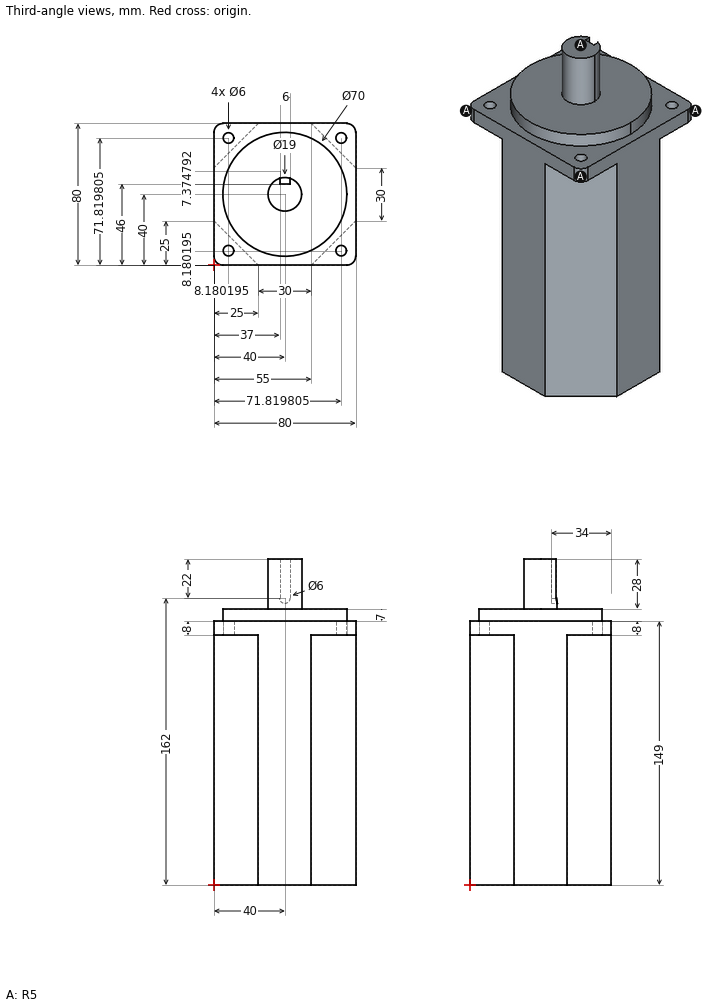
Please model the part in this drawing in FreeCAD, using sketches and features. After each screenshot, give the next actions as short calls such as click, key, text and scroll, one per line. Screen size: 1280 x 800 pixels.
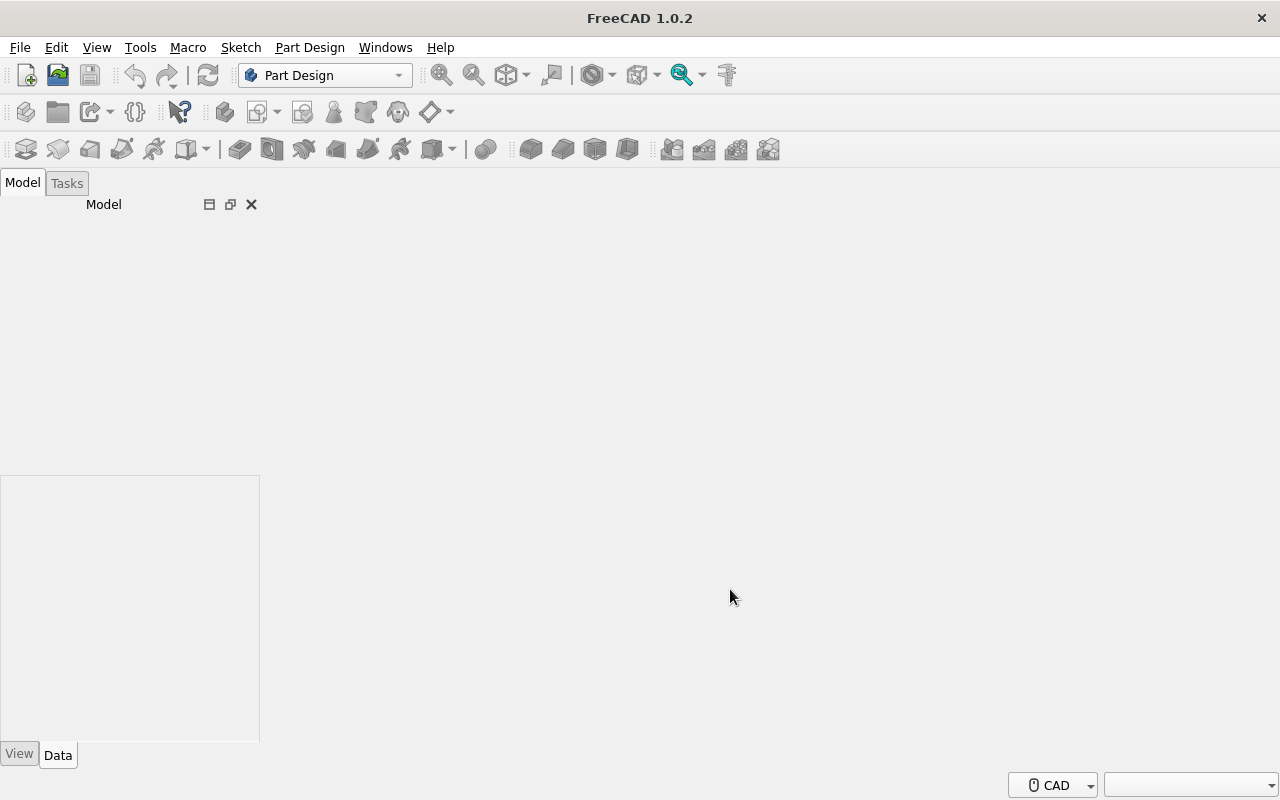
key(ctrl+n)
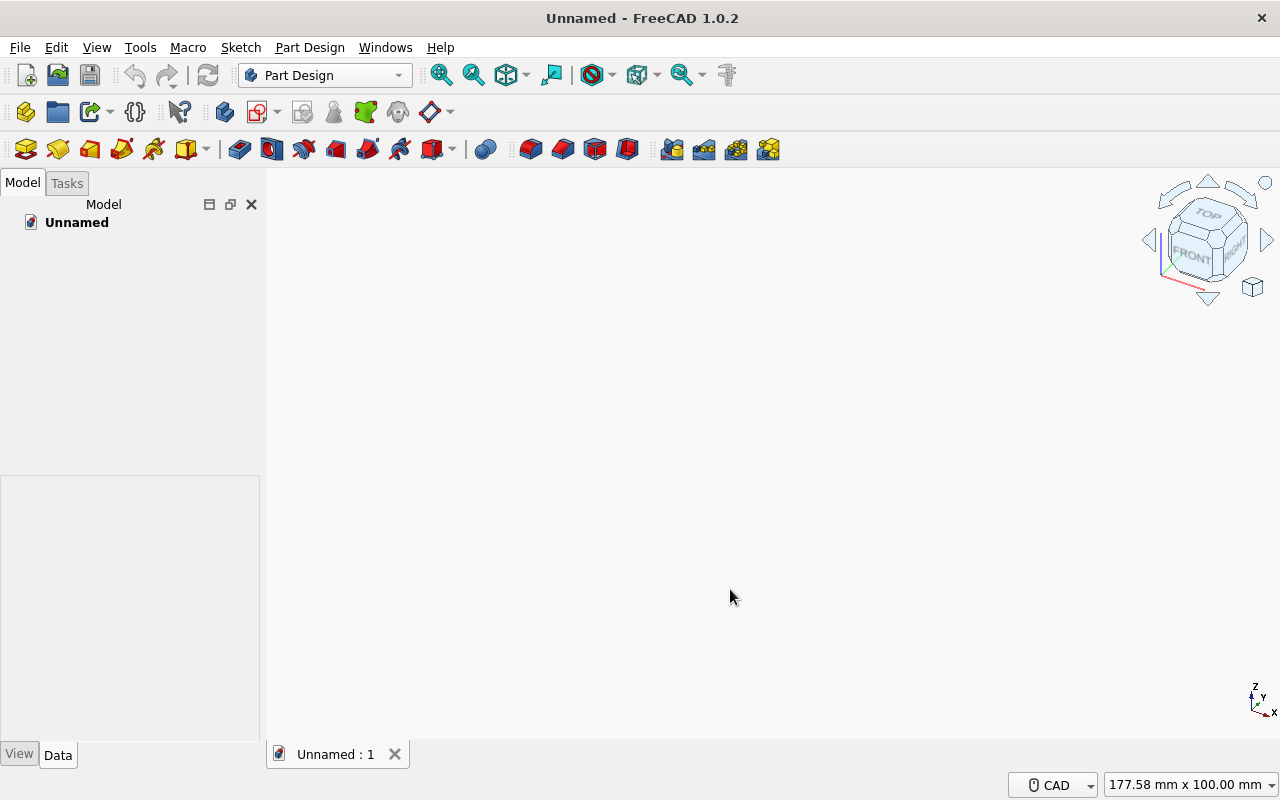
click(258, 112)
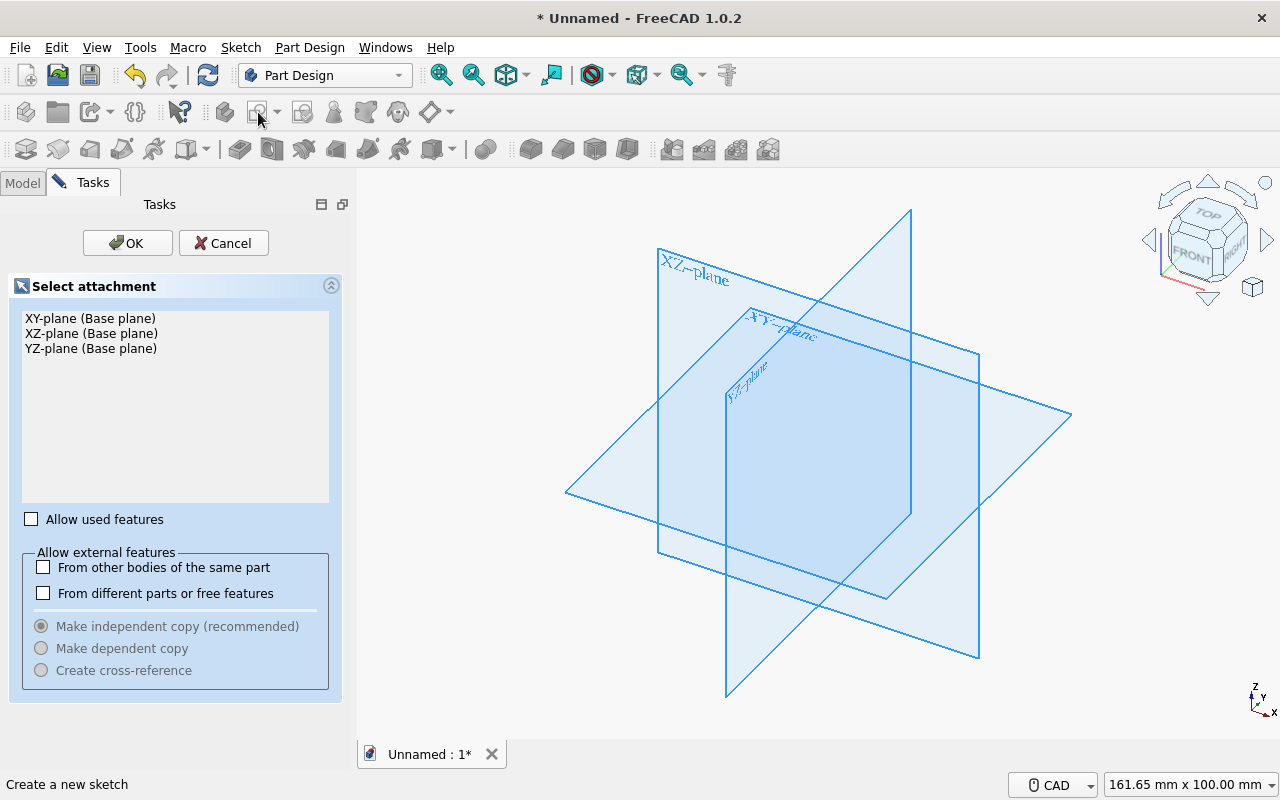
click(82, 318)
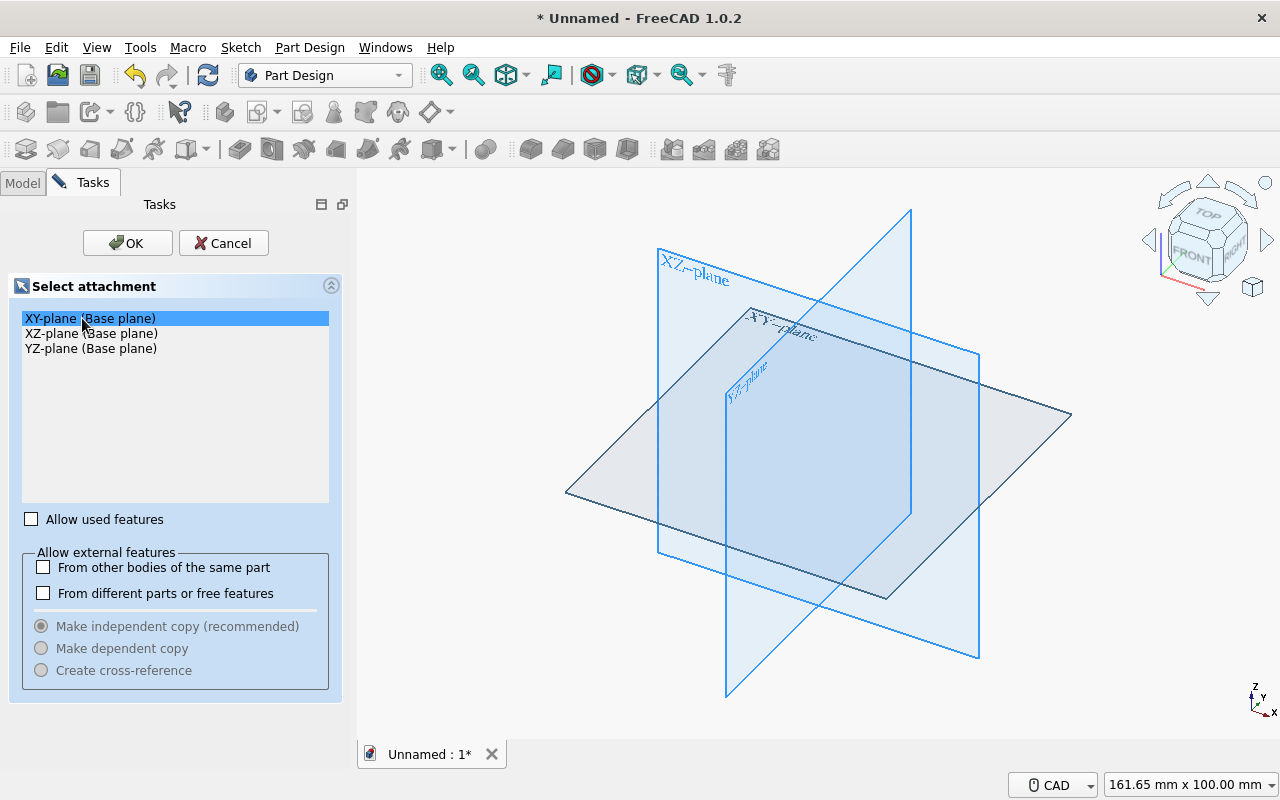
click(128, 243)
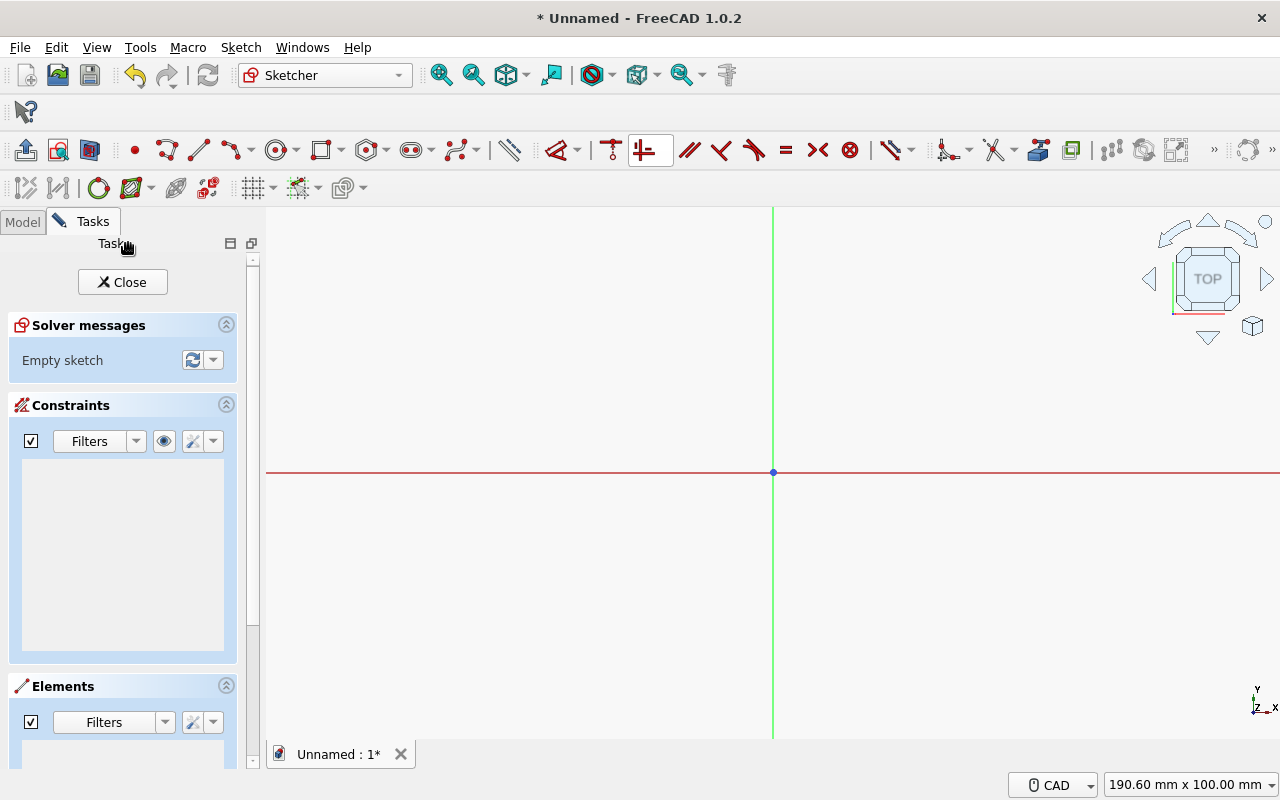
scroll(294, 711, down, 2)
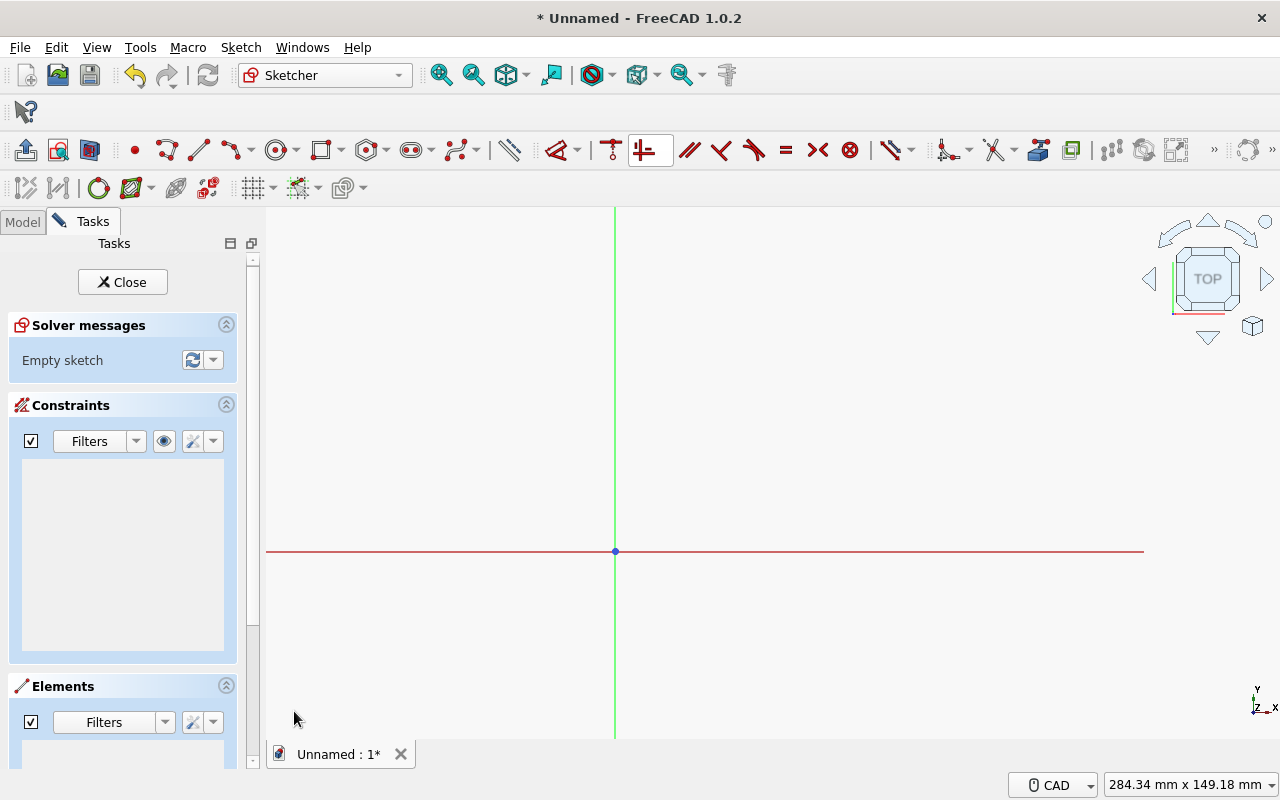
key(g)
key(m)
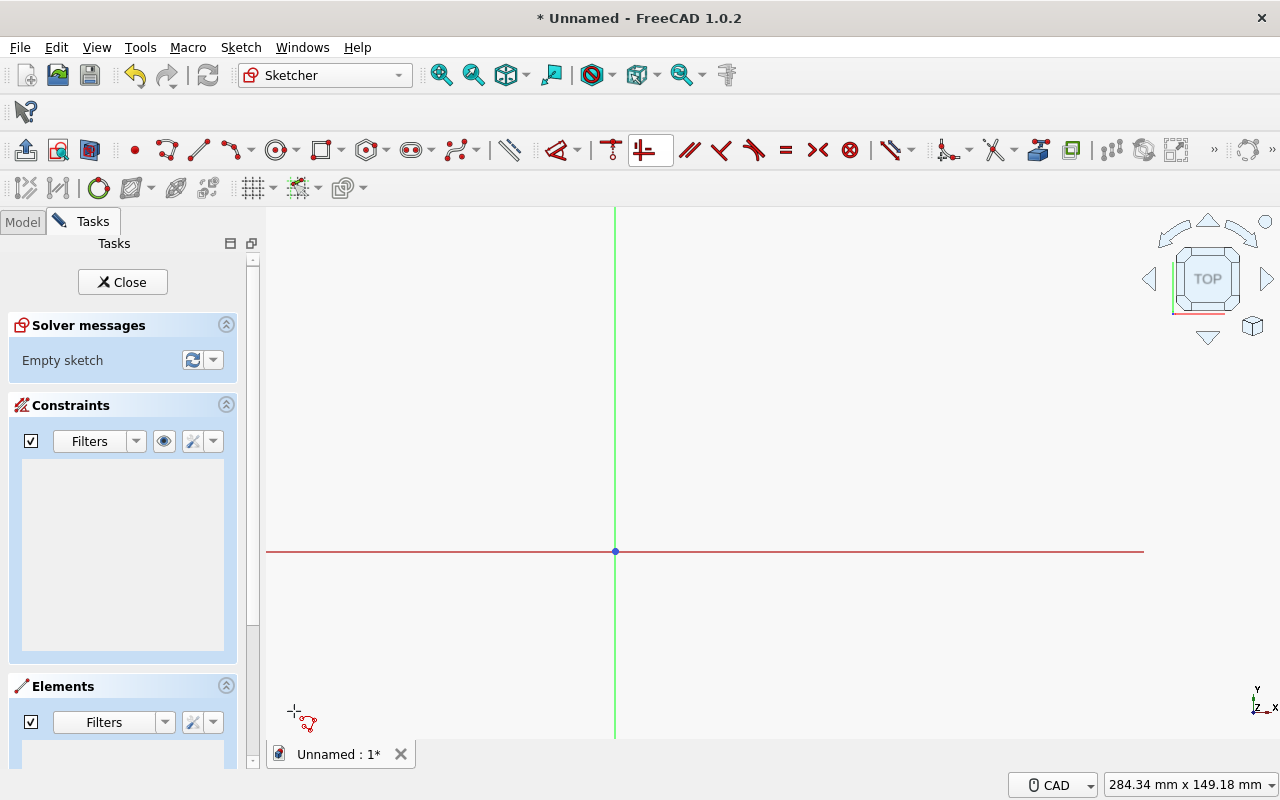
click(615, 463)
click(704, 552)
click(811, 543)
click(900, 463)
click(900, 356)
click(811, 266)
click(704, 266)
click(624, 356)
click(615, 464)
key(Escape)
key(Escape)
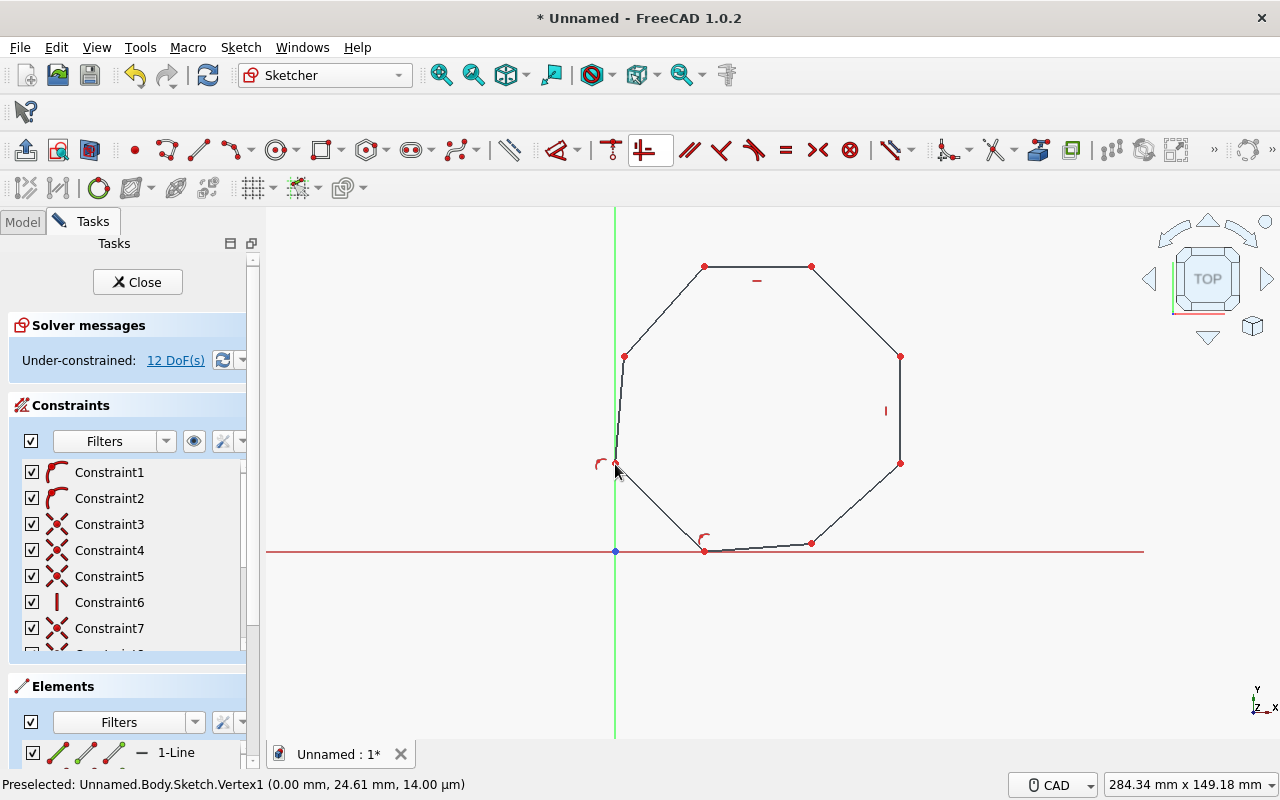
click(736, 549)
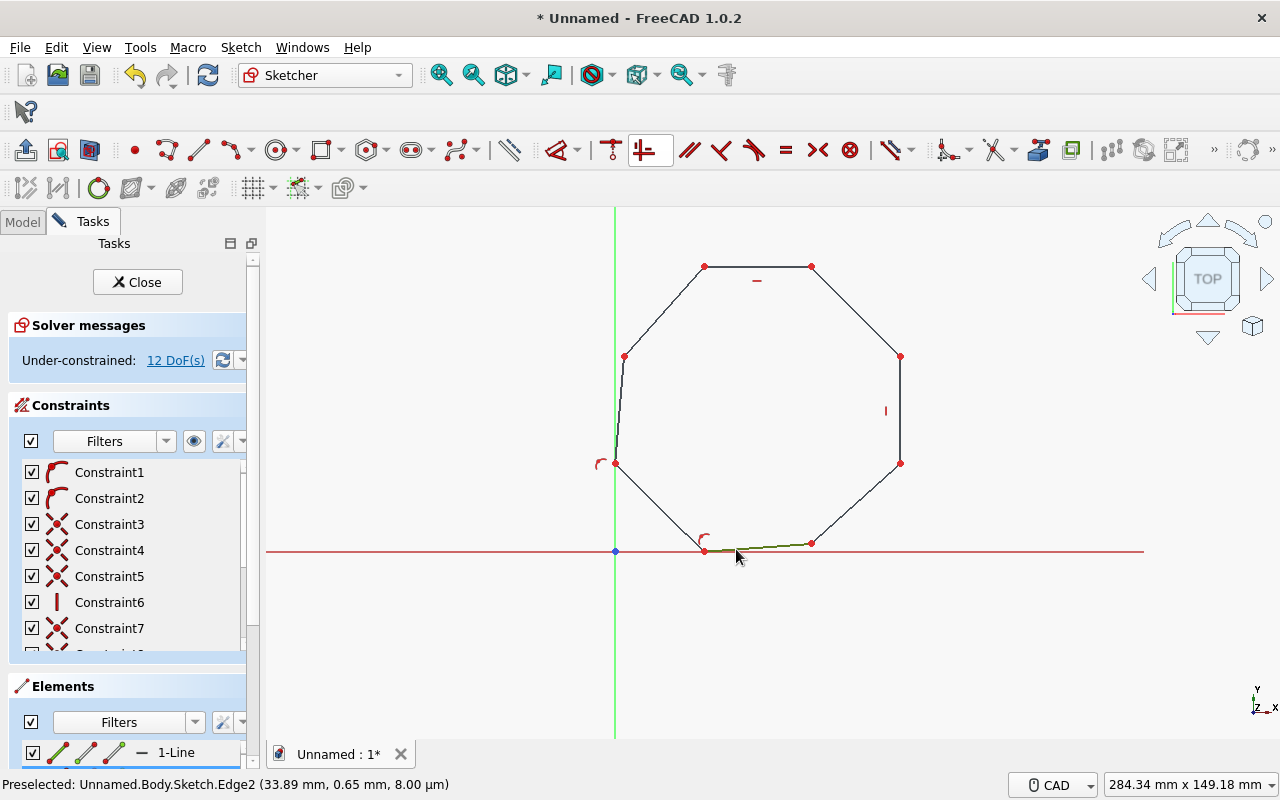
key(h)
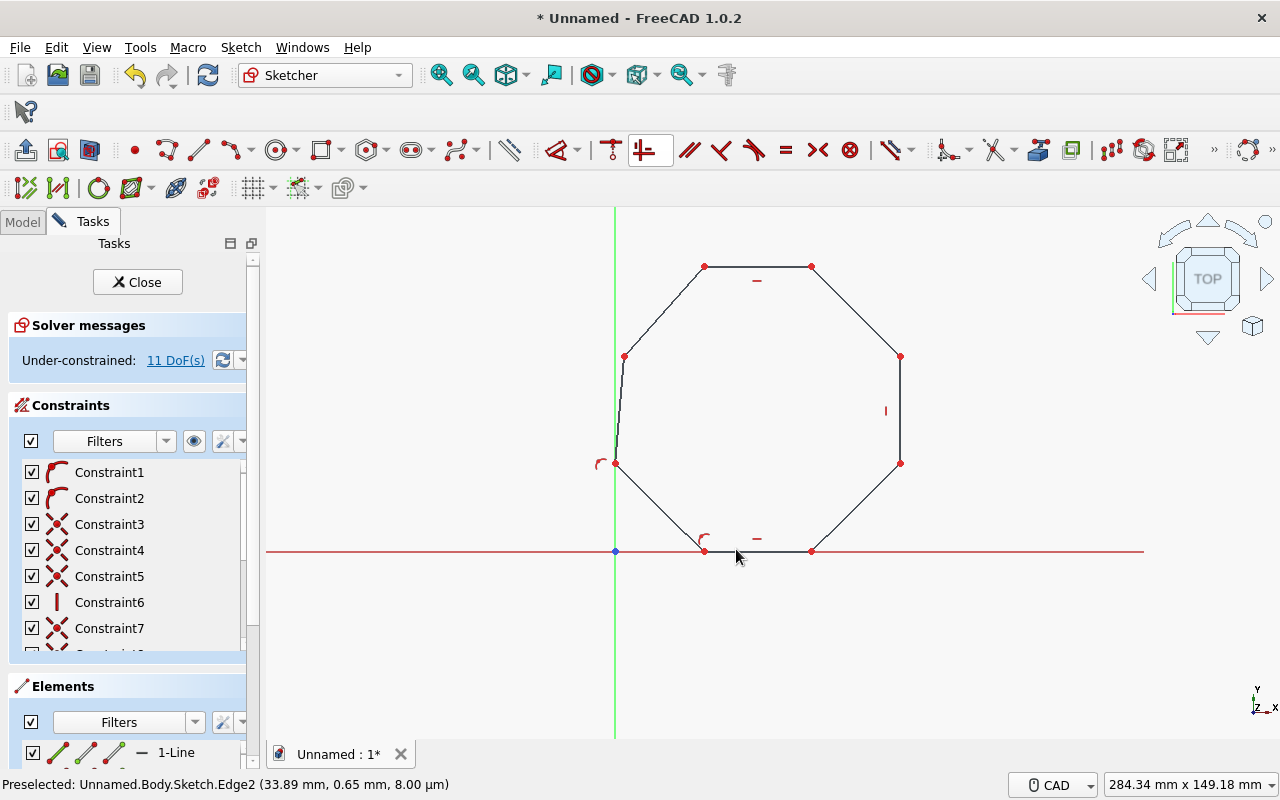
click(618, 432)